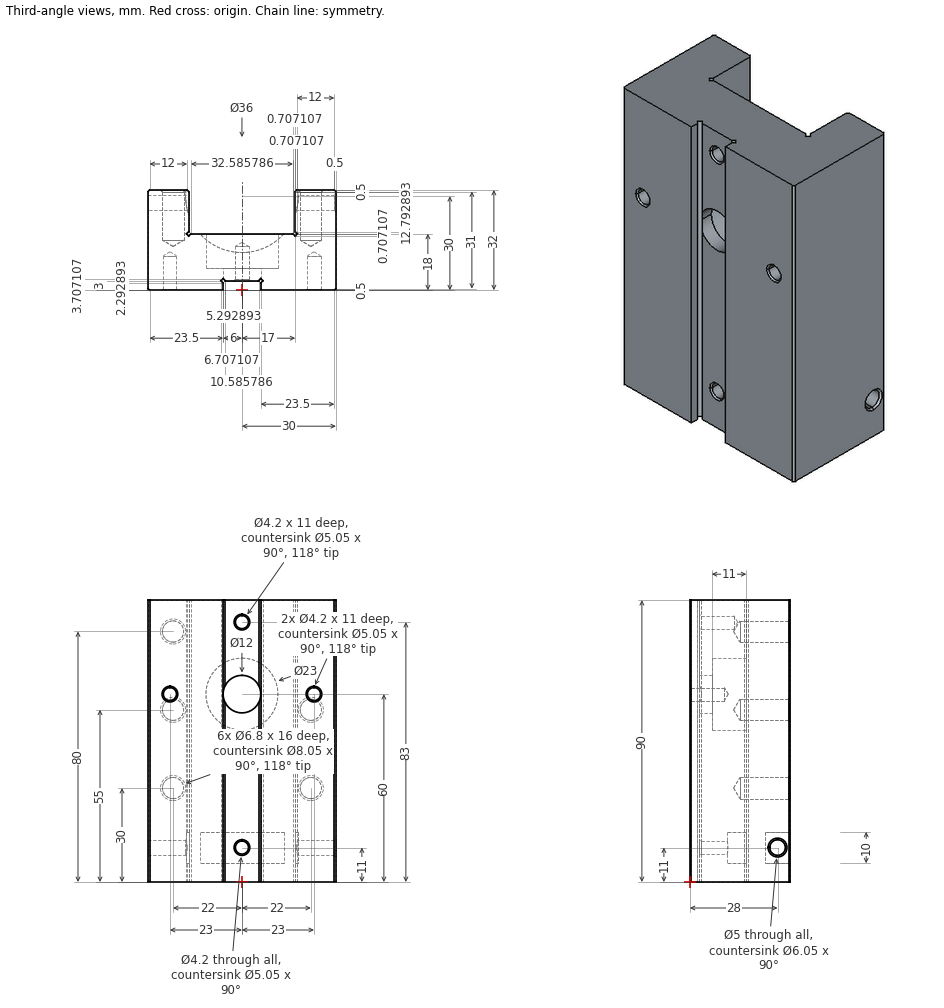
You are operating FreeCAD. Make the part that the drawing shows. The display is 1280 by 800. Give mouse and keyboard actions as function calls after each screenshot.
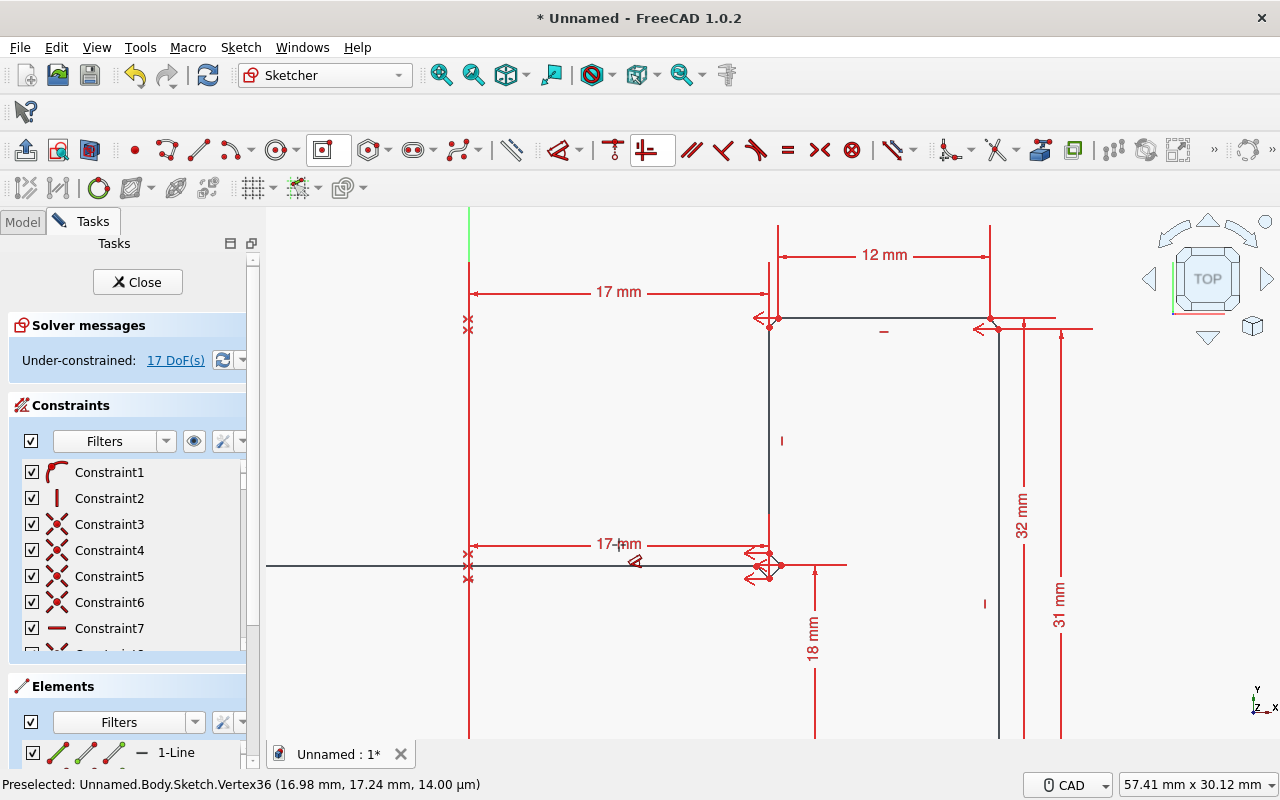
click(757, 566)
click(791, 605)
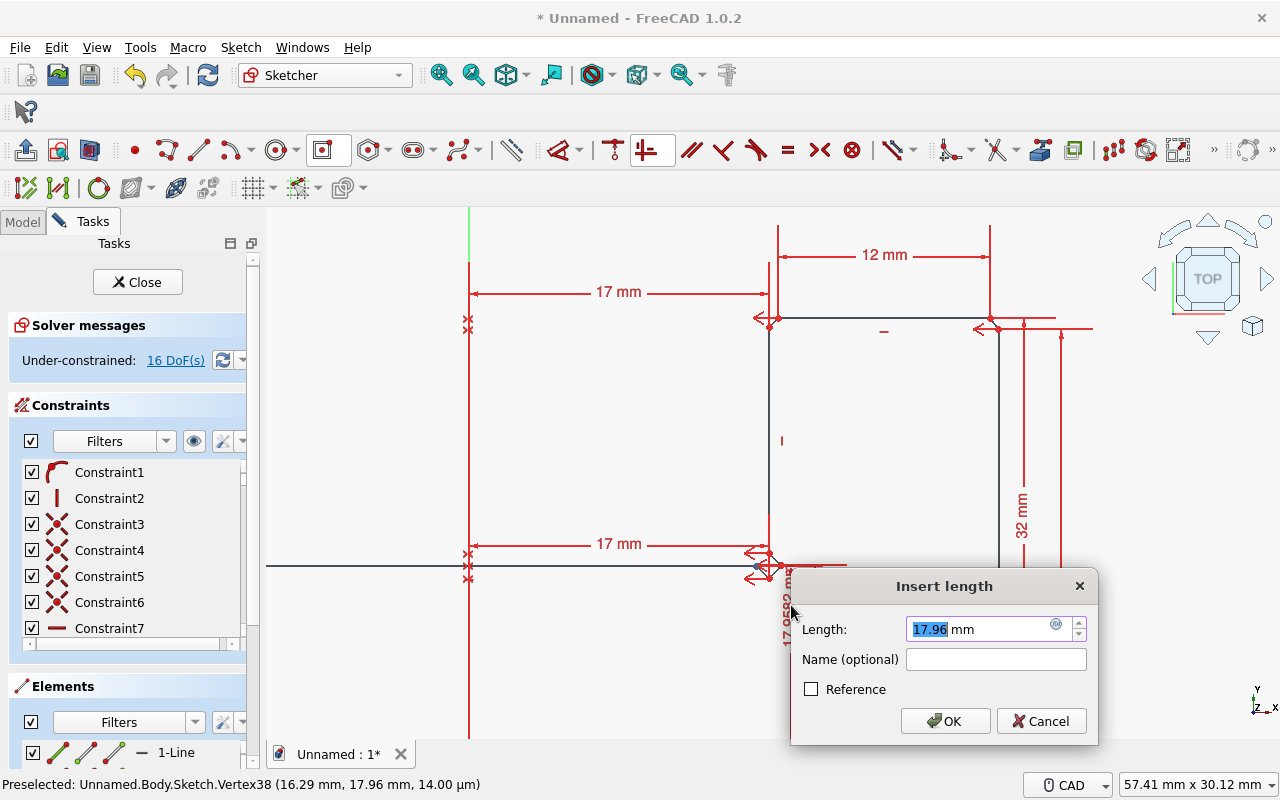
text(18)
key(Return)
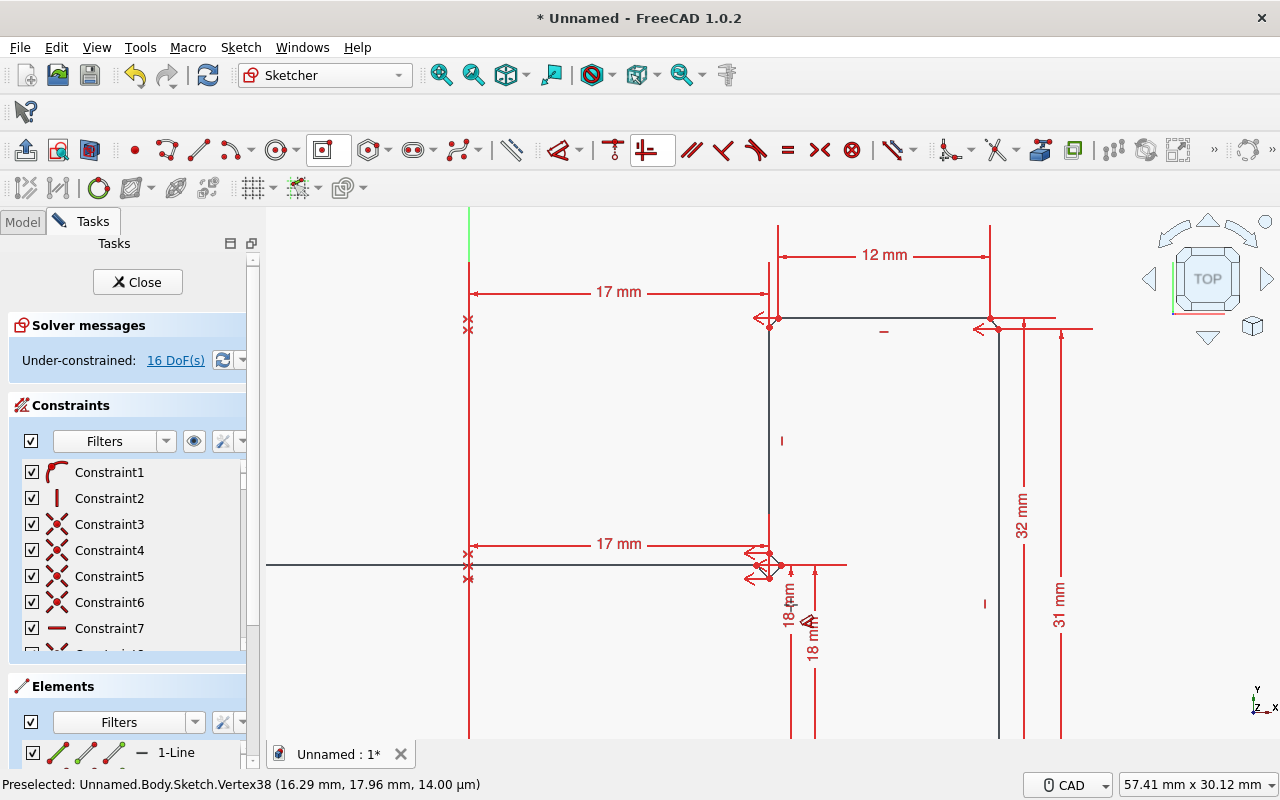
scroll(991, 318, down, 3)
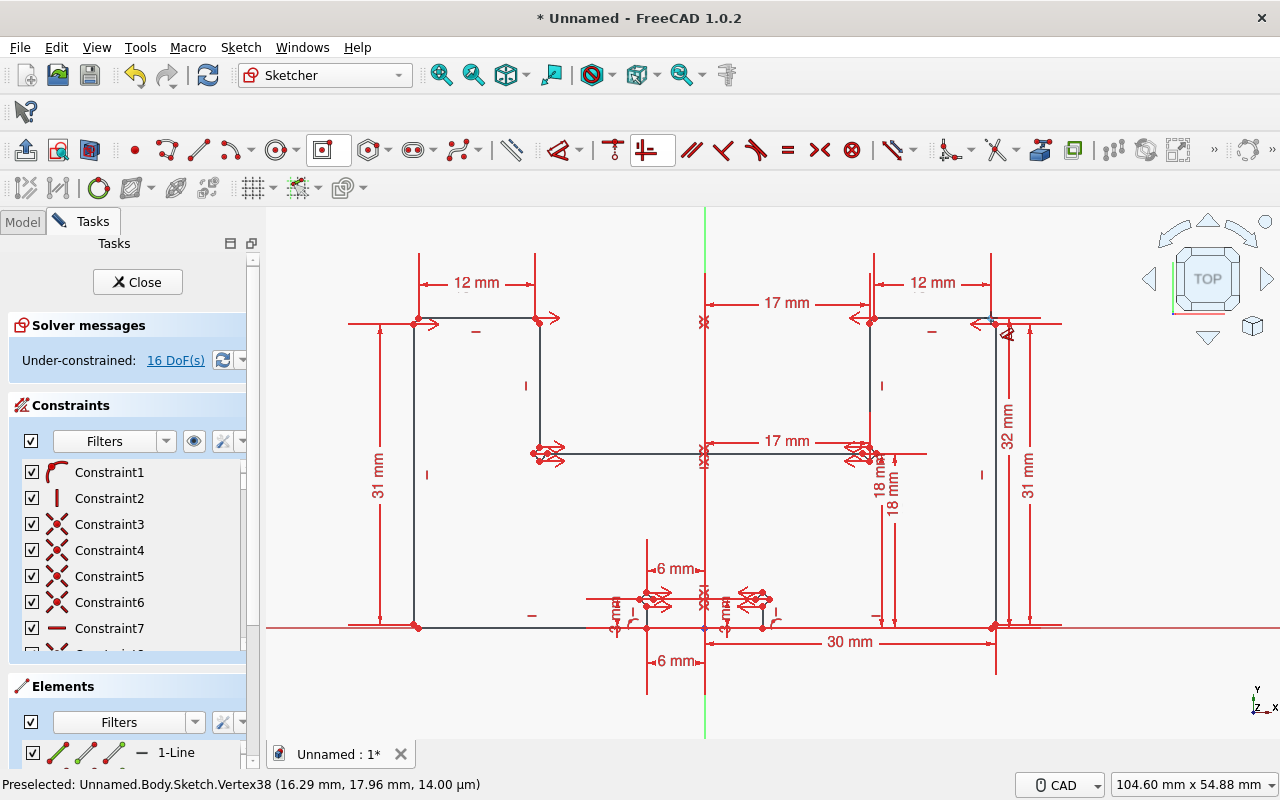
click(831, 628)
click(929, 662)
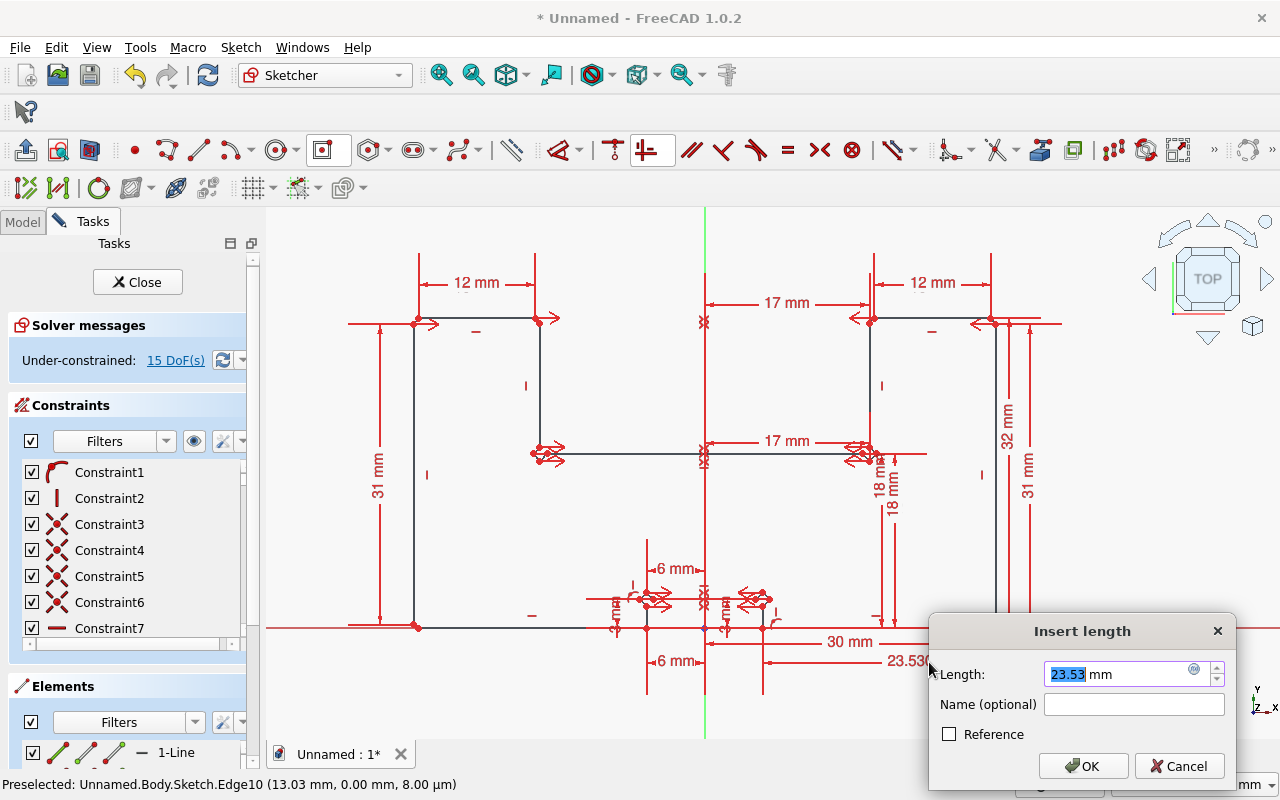
text(23.5)
key(Return)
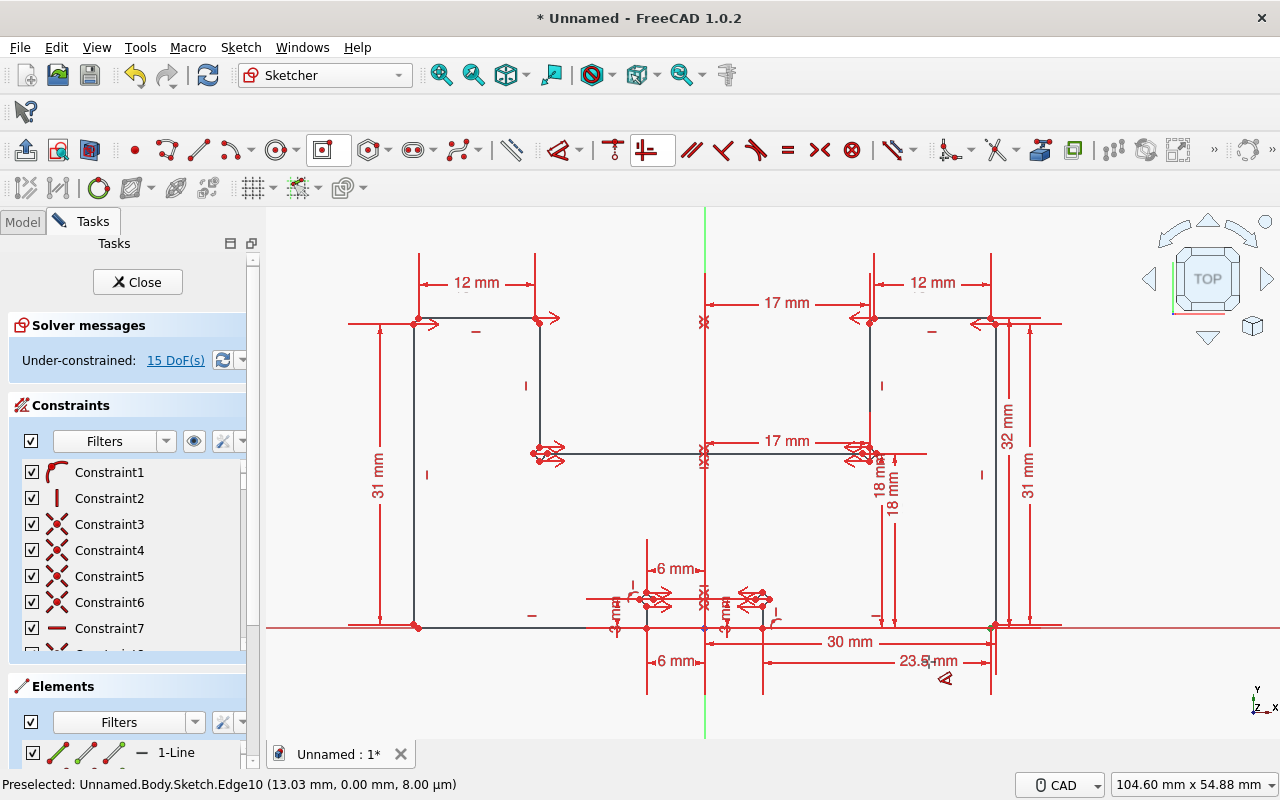
click(487, 628)
click(533, 662)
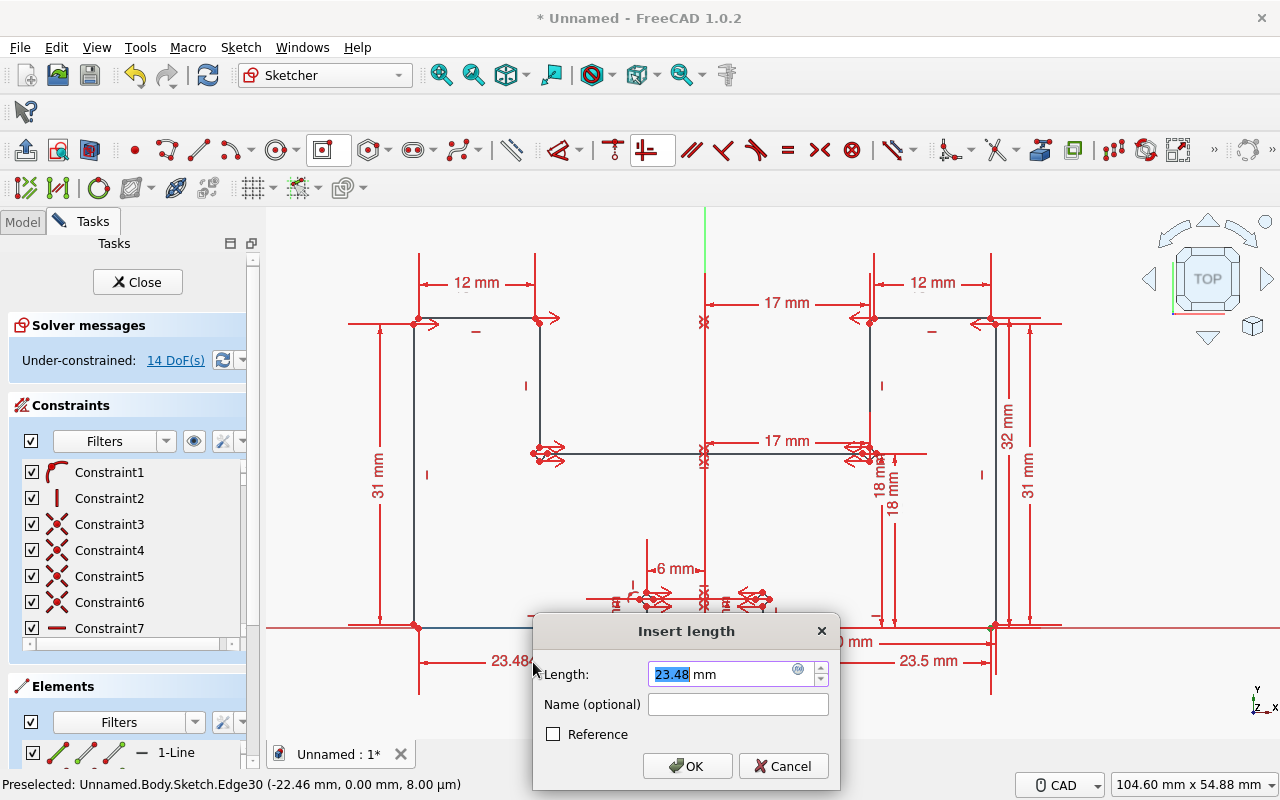
text(23.5)
key(Return)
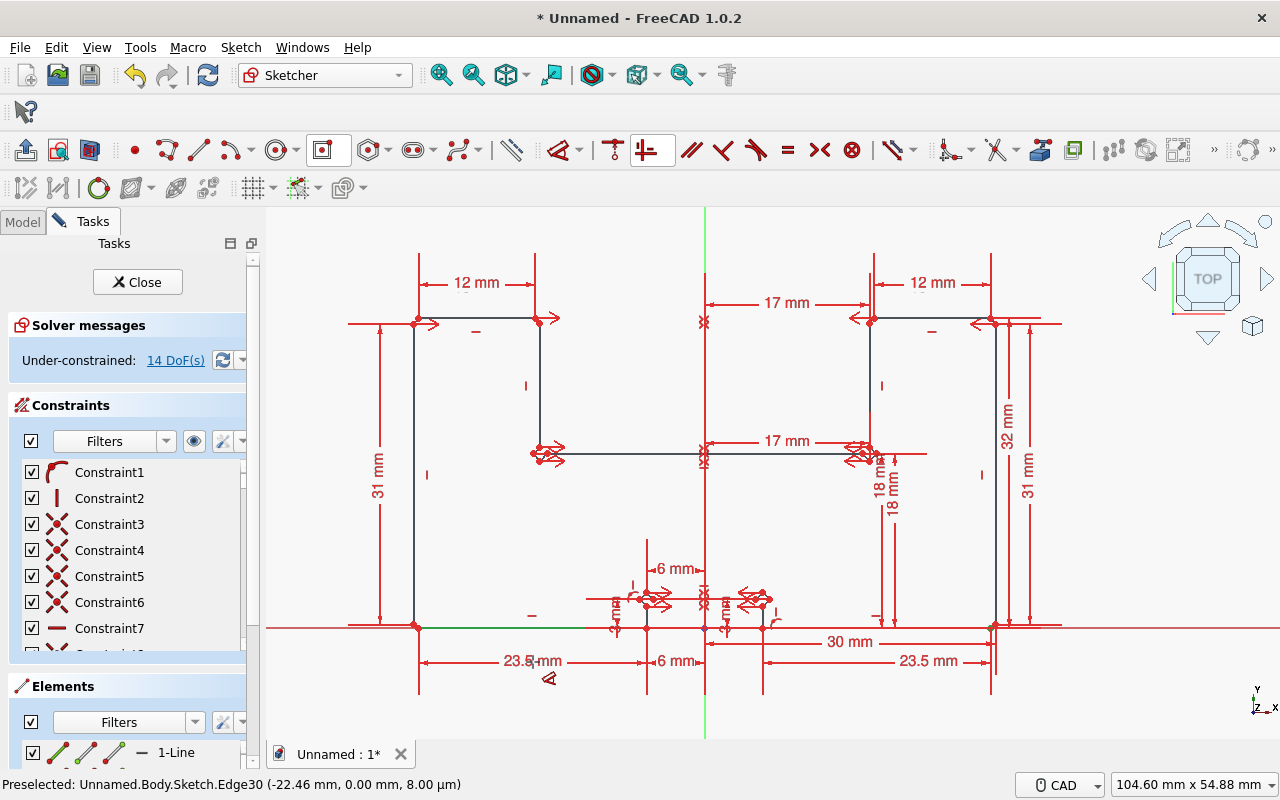
scroll(996, 625, up, 11)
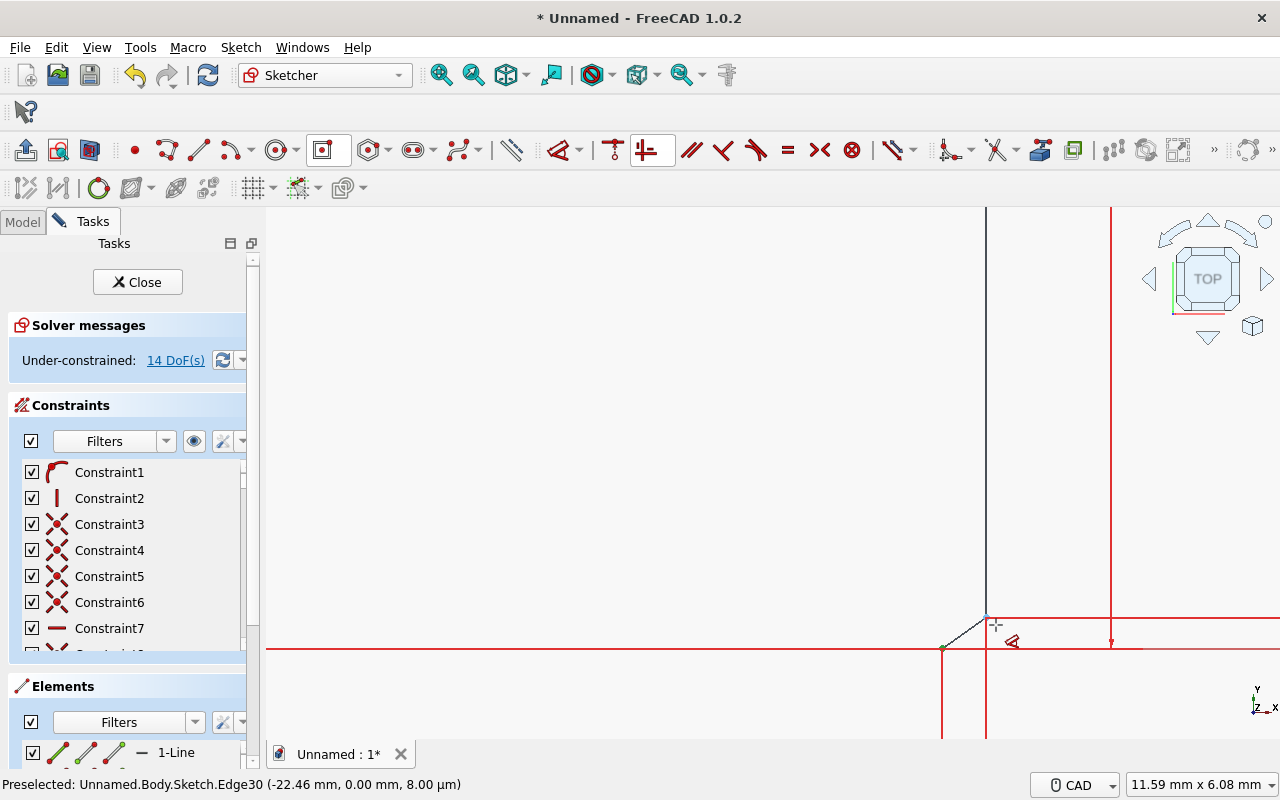
click(986, 618)
click(1020, 633)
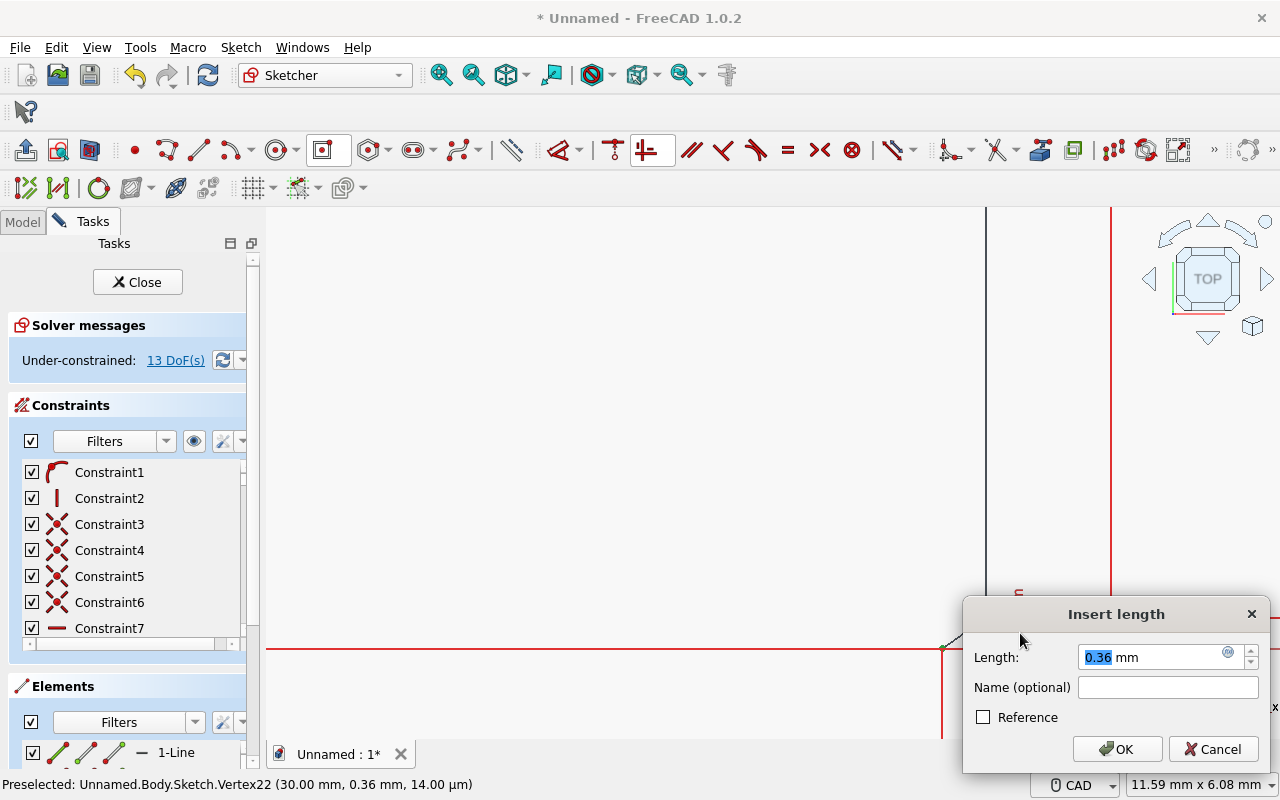
text(0.5)
key(Return)